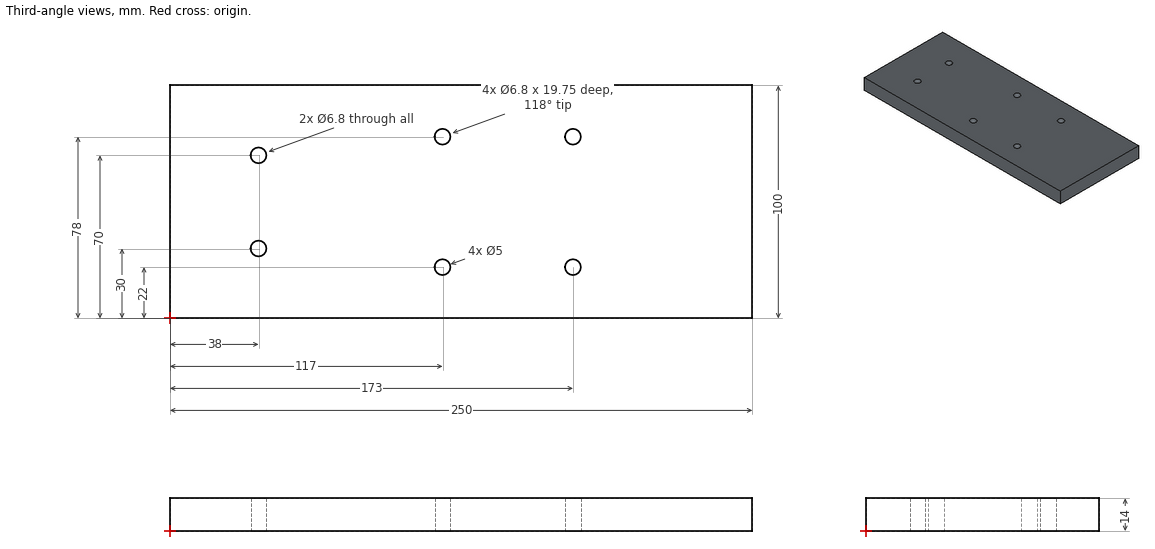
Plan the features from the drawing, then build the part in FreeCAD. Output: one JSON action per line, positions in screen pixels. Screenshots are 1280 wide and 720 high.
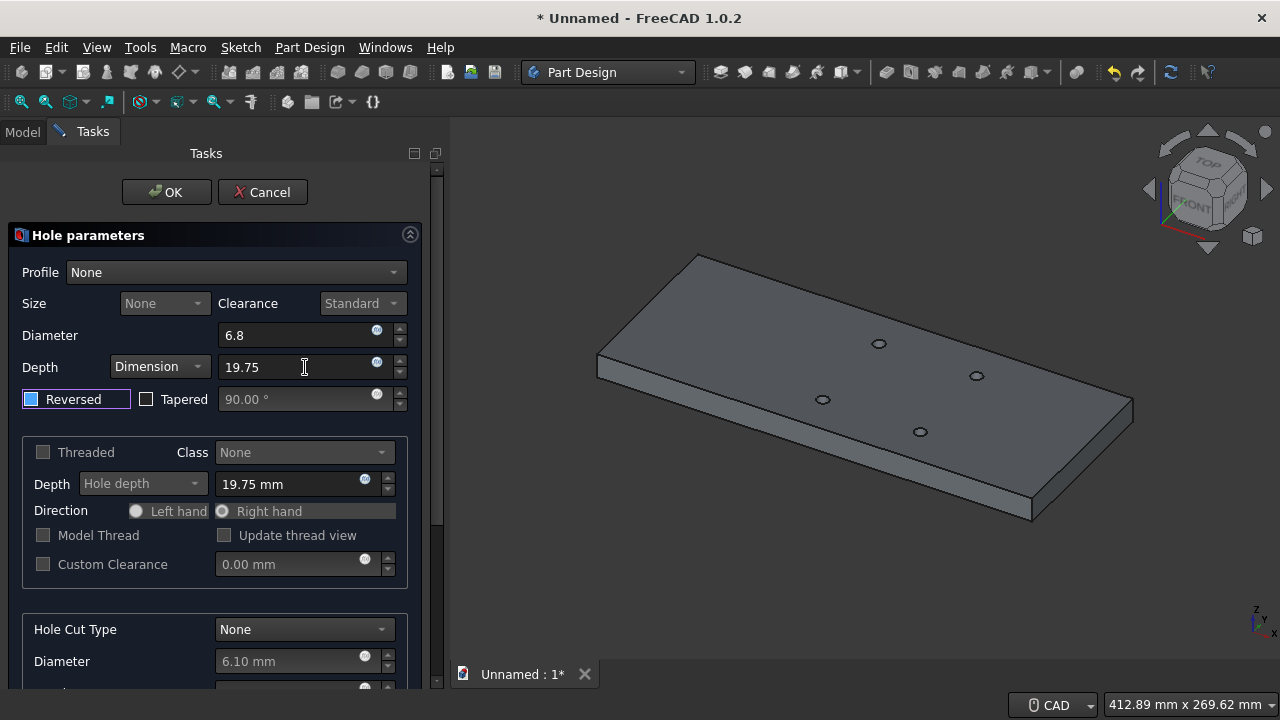
{"action": "left_click", "coordinate": [167, 192]}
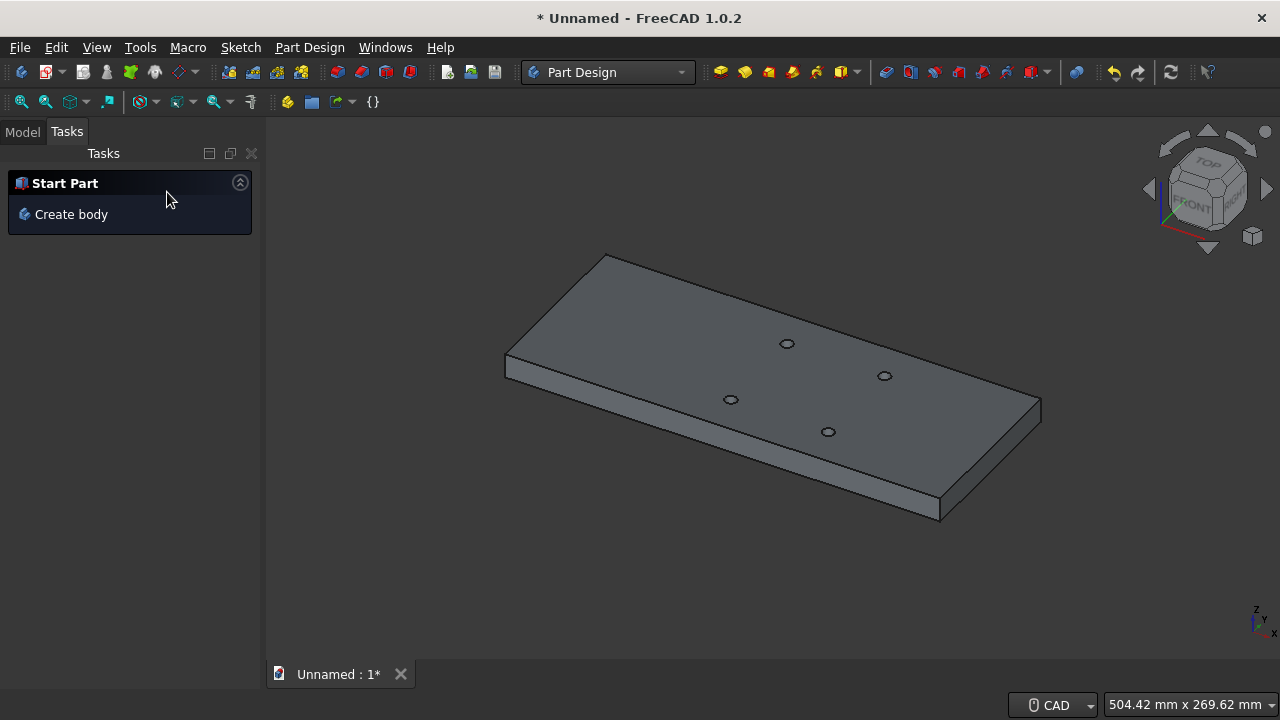
{"action": "left_click", "coordinate": [649, 334]}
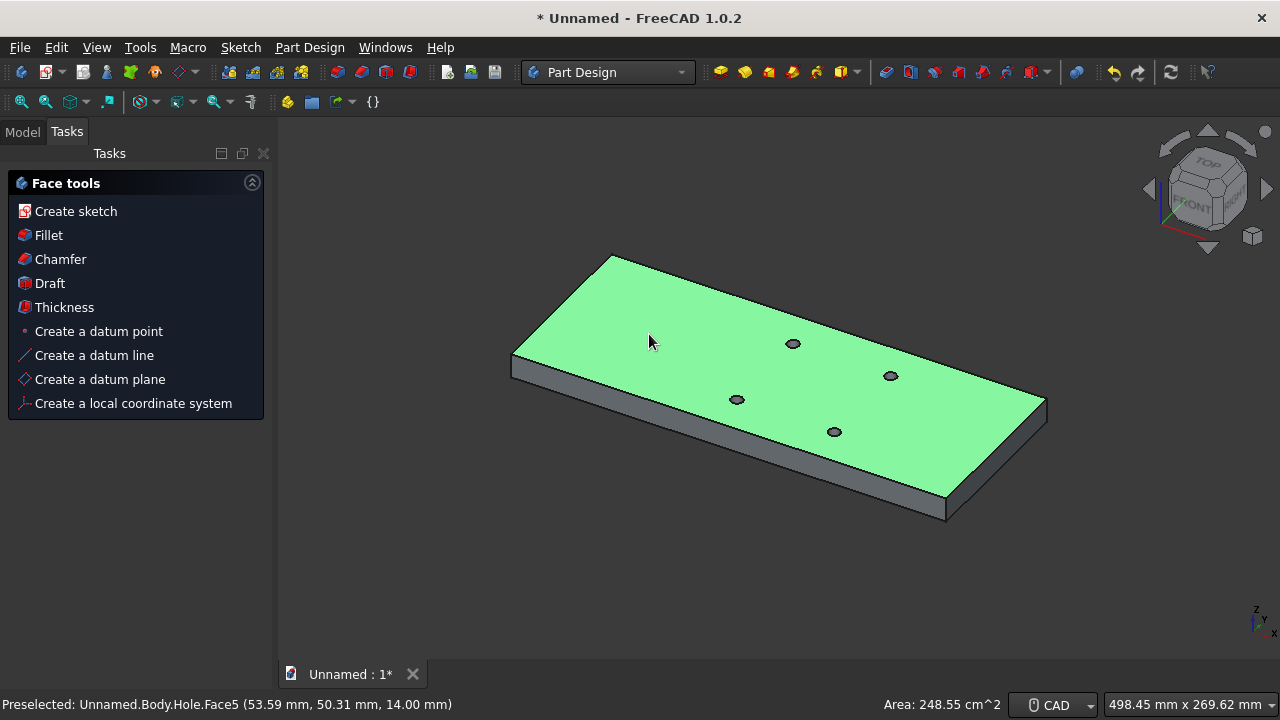
{"action": "left_click", "coordinate": [46, 72]}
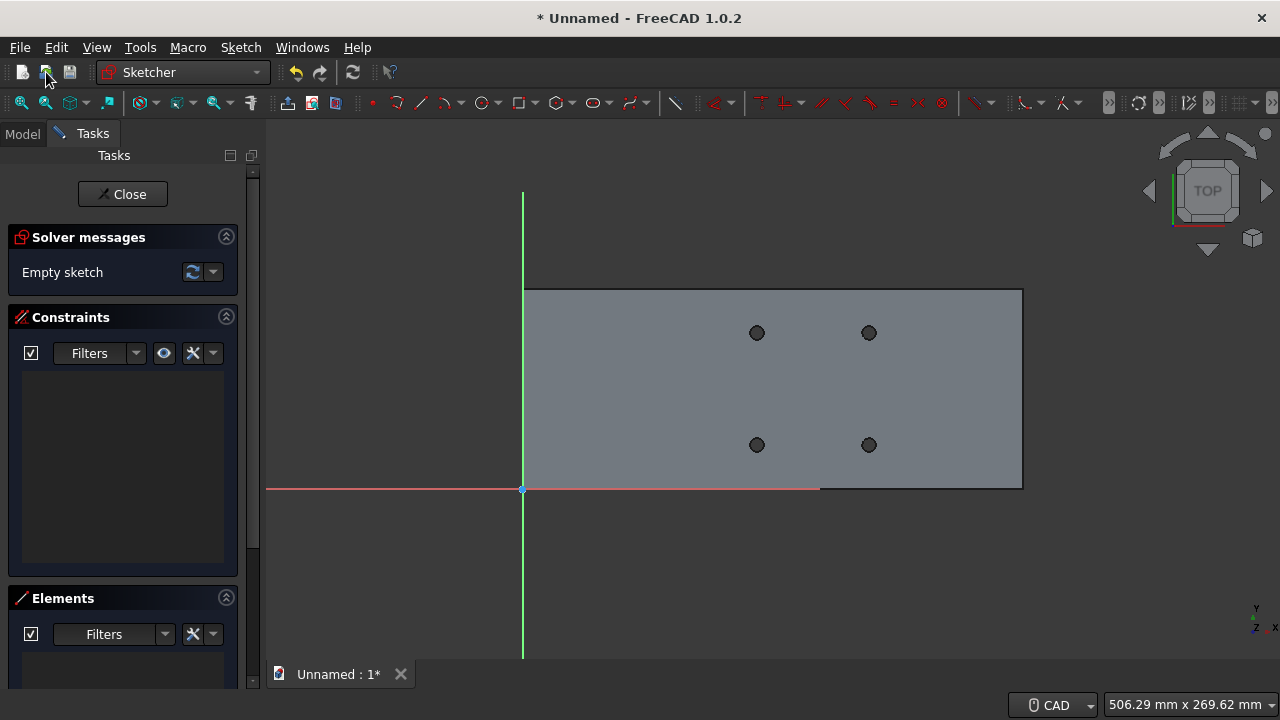
{"action": "scroll", "coordinate": [450, 437], "scroll_direction": "up", "scroll_amount": 4}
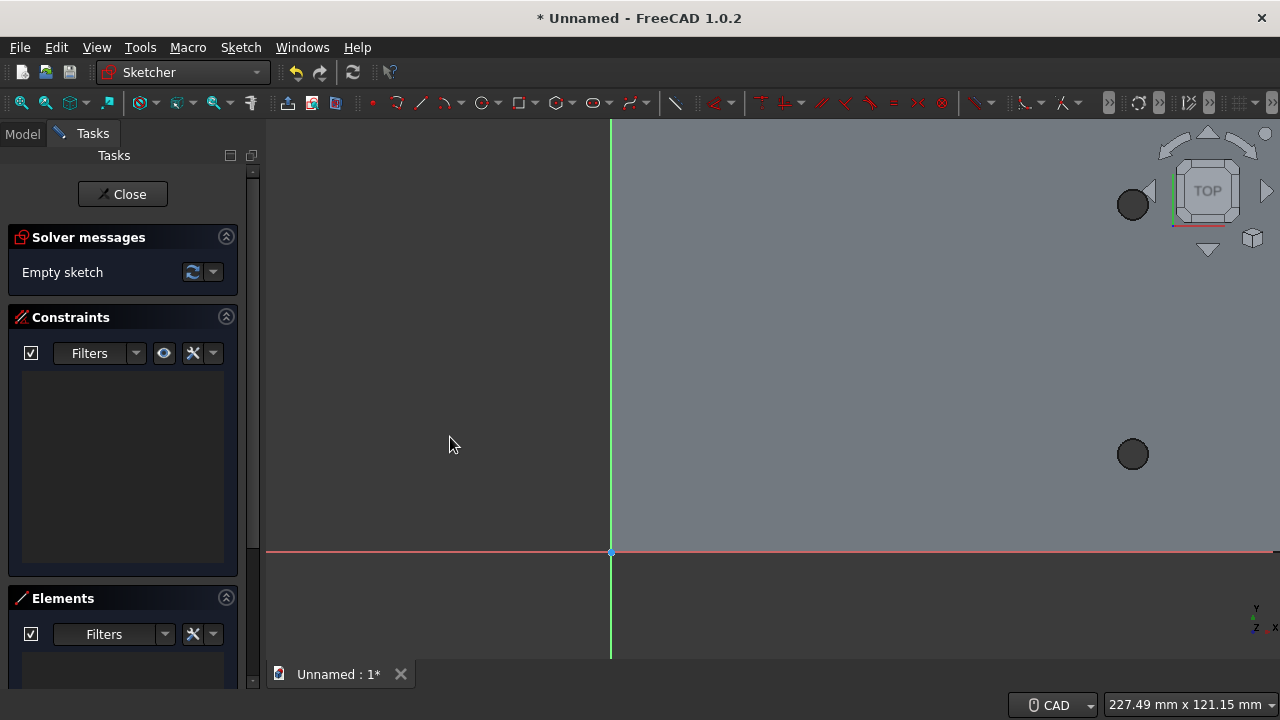
{"action": "left_click", "coordinate": [482, 104]}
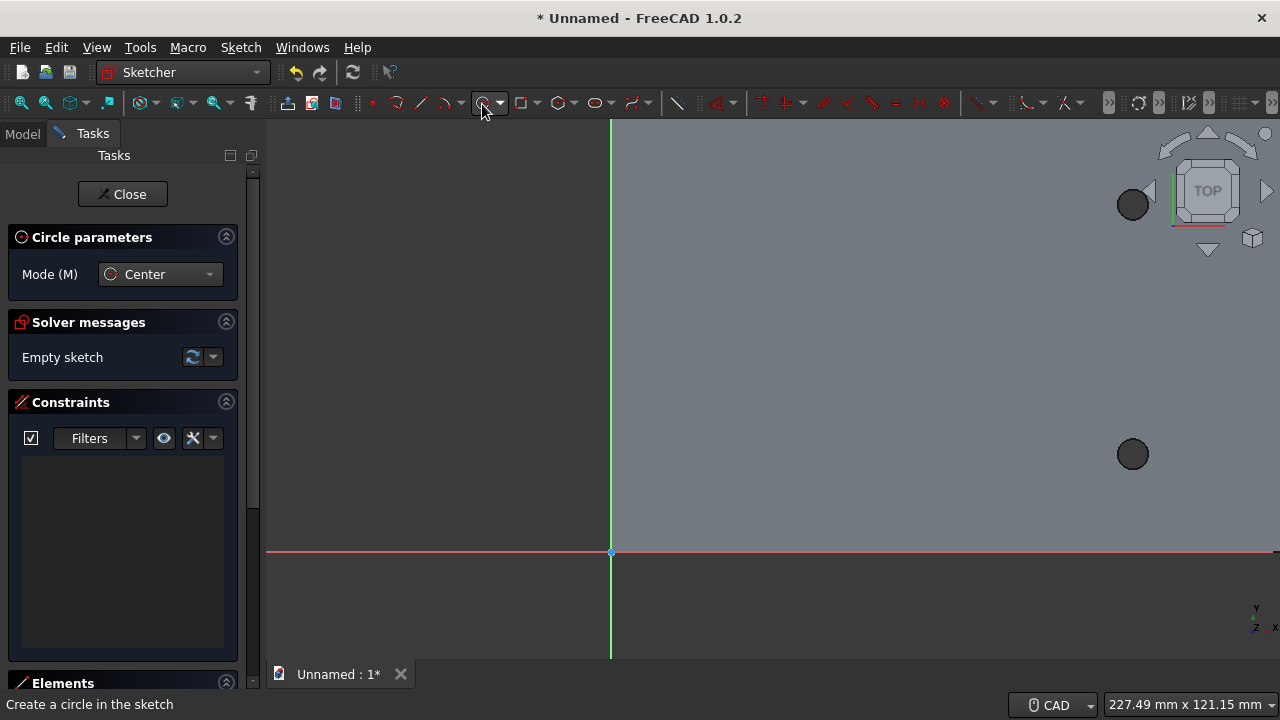
{"action": "scroll", "coordinate": [781, 240], "scroll_direction": "up", "scroll_amount": 3}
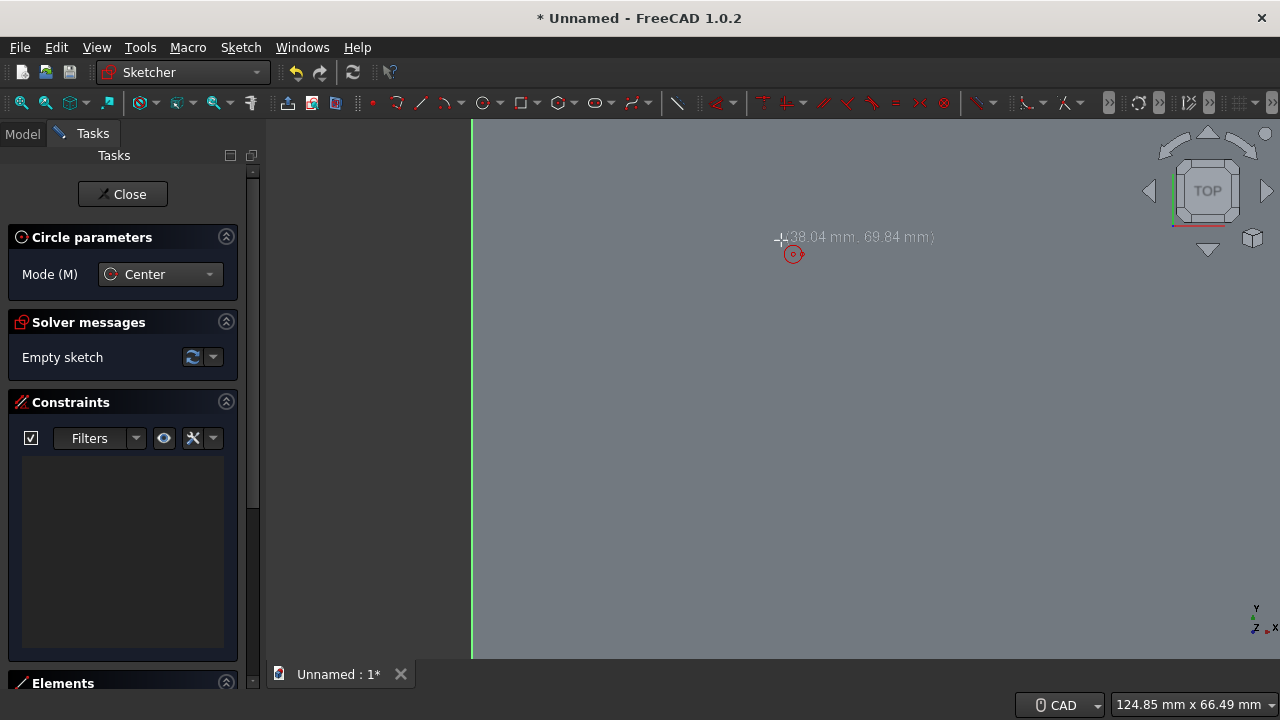
{"action": "left_click", "coordinate": [780, 240]}
{"action": "left_click", "coordinate": [800, 221]}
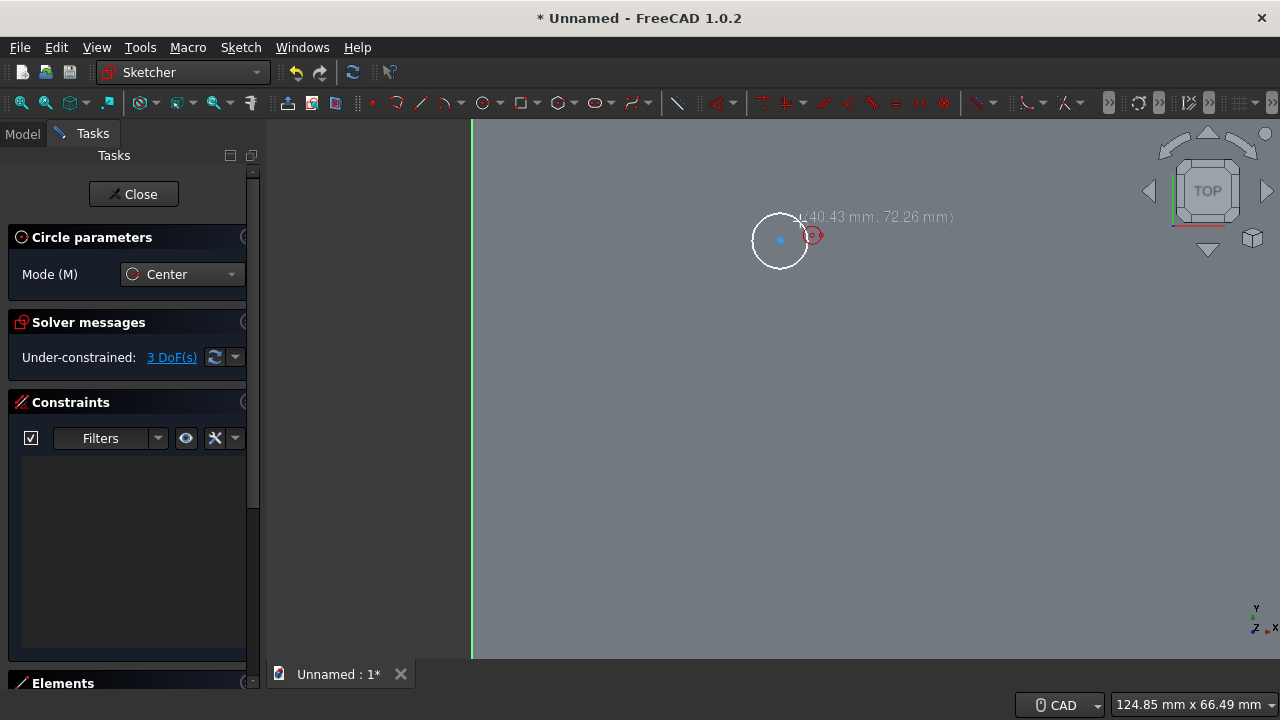
{"action": "left_click", "coordinate": [780, 565]}
{"action": "left_click", "coordinate": [800, 546]}
{"action": "key", "text": "Escape"}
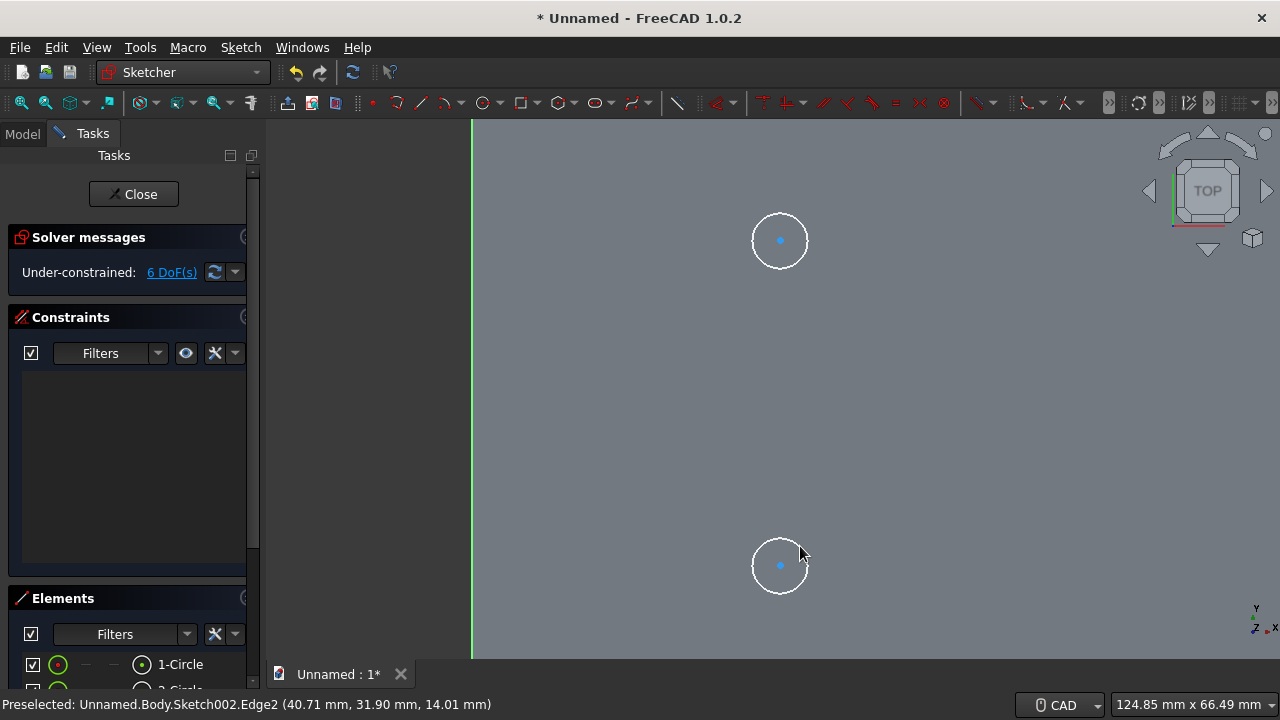
{"action": "left_click", "coordinate": [799, 221]}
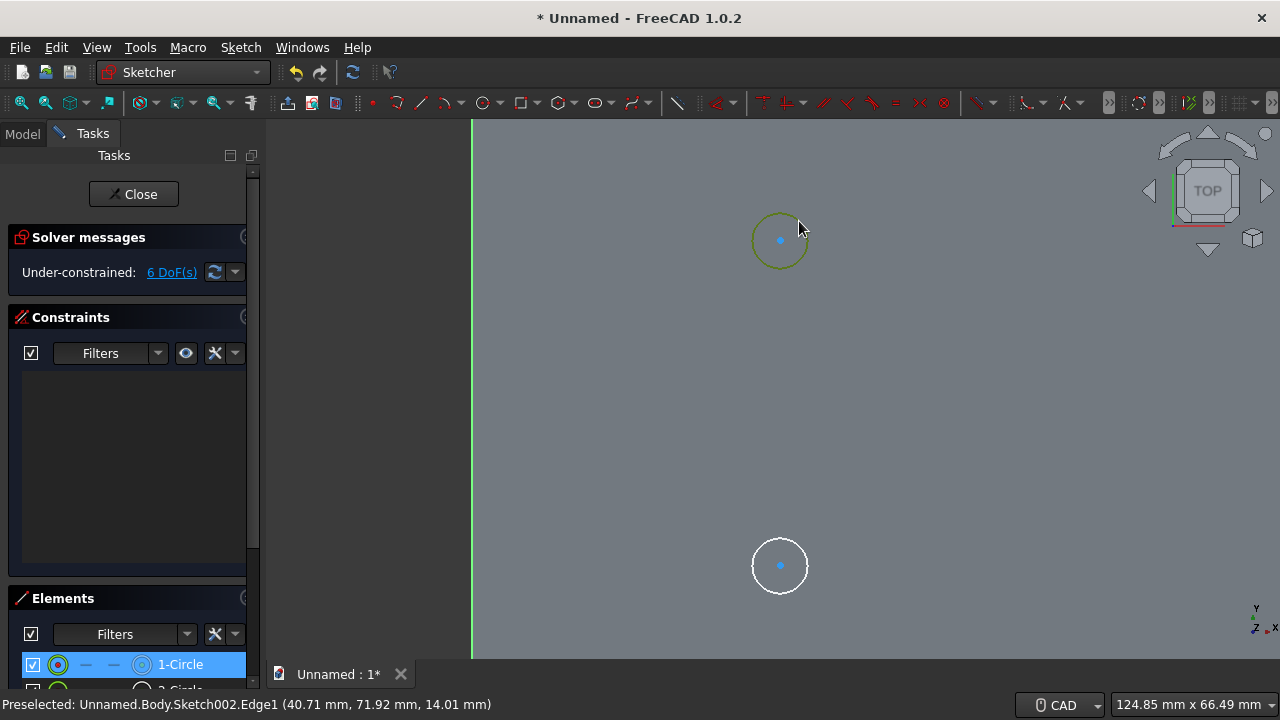
{"action": "left_click", "coordinate": [799, 546]}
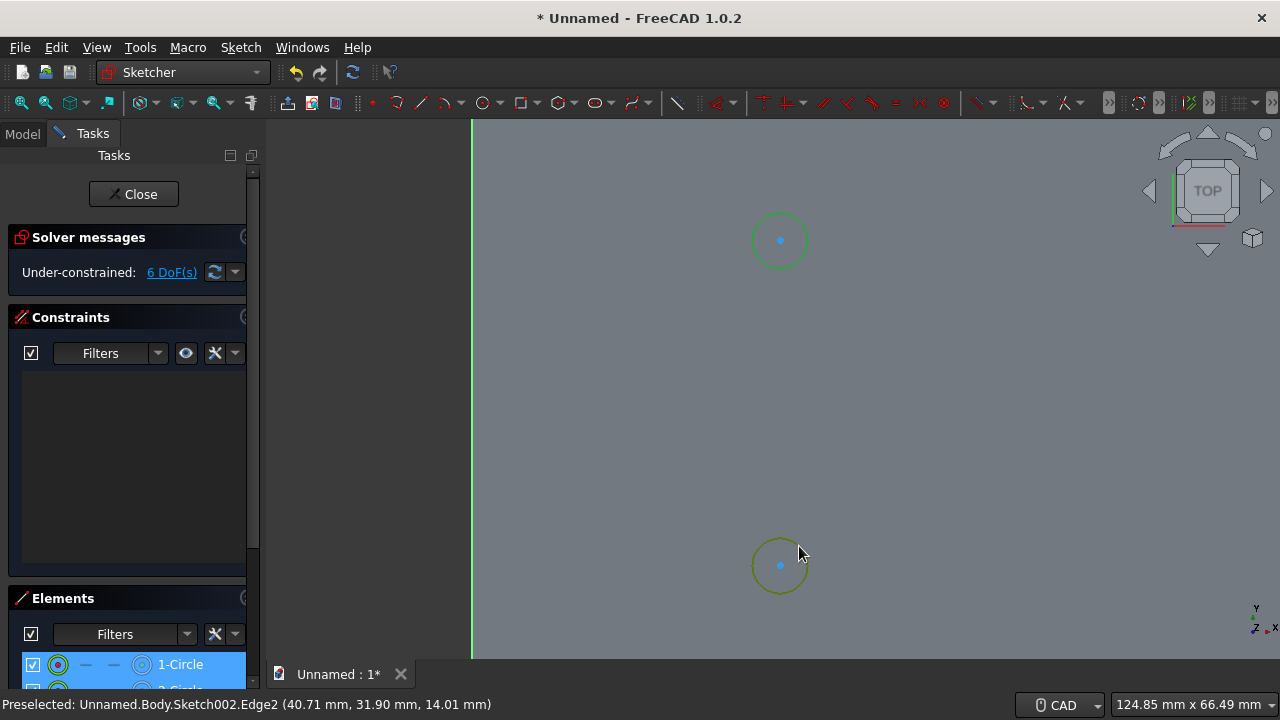
{"action": "left_click", "coordinate": [896, 104]}